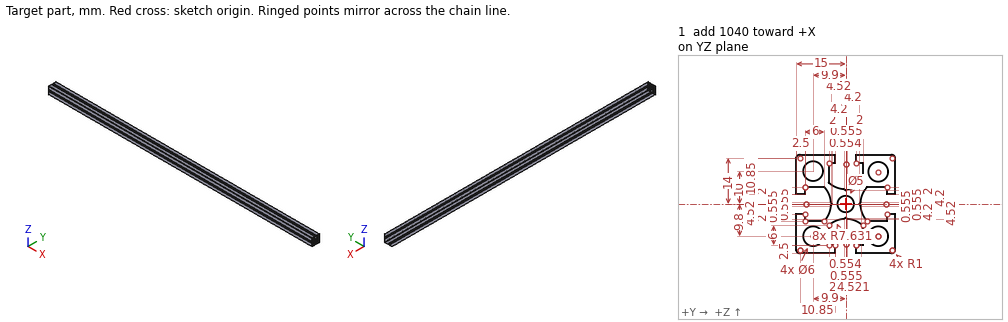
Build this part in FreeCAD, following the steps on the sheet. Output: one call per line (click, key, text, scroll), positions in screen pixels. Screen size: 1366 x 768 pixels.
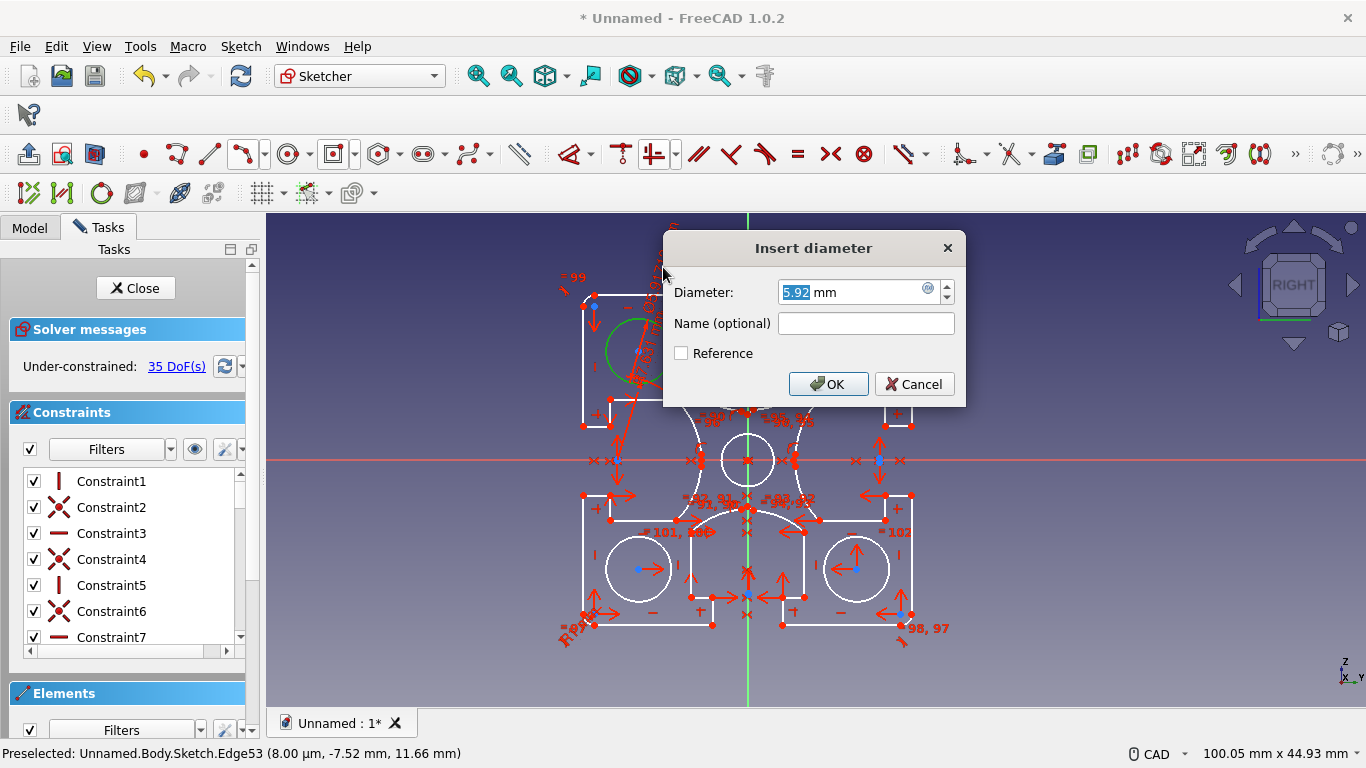
text(6)
key(Return)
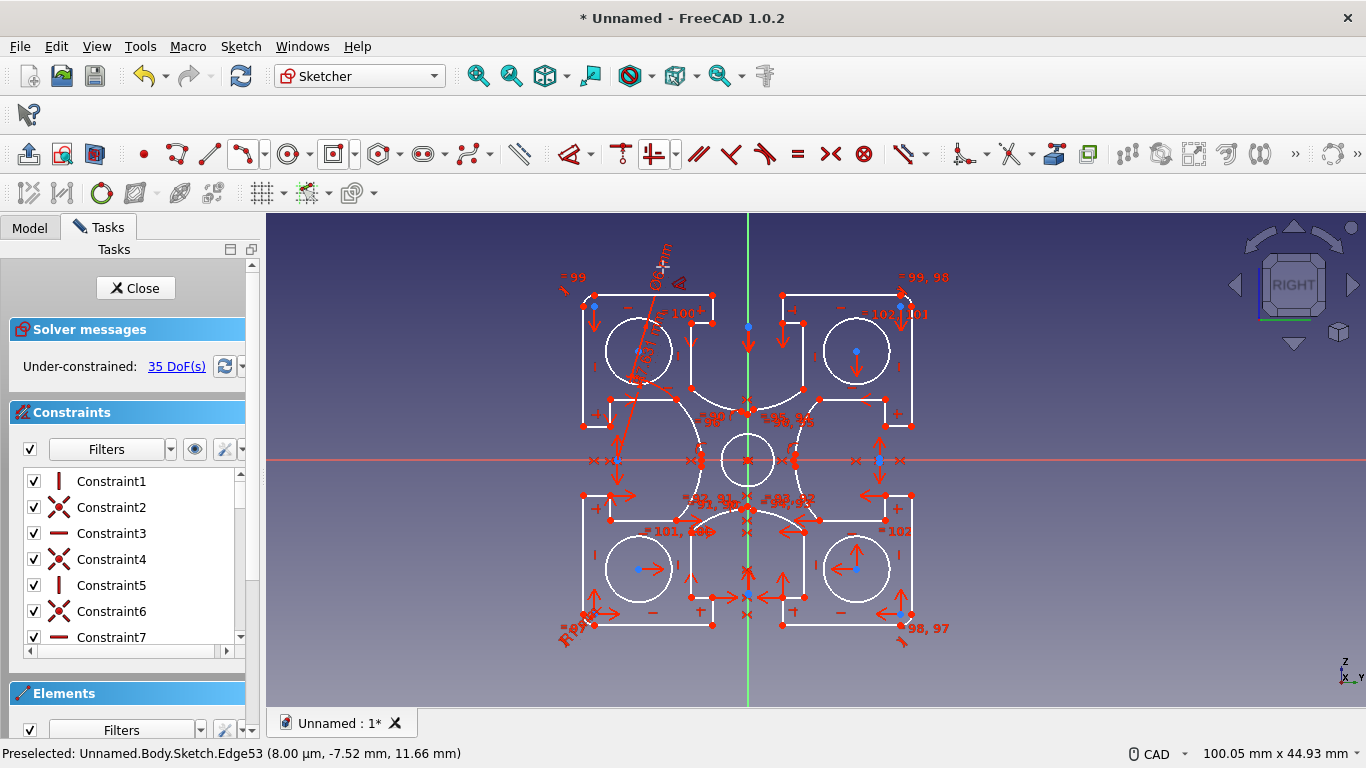
click(766, 442)
click(789, 419)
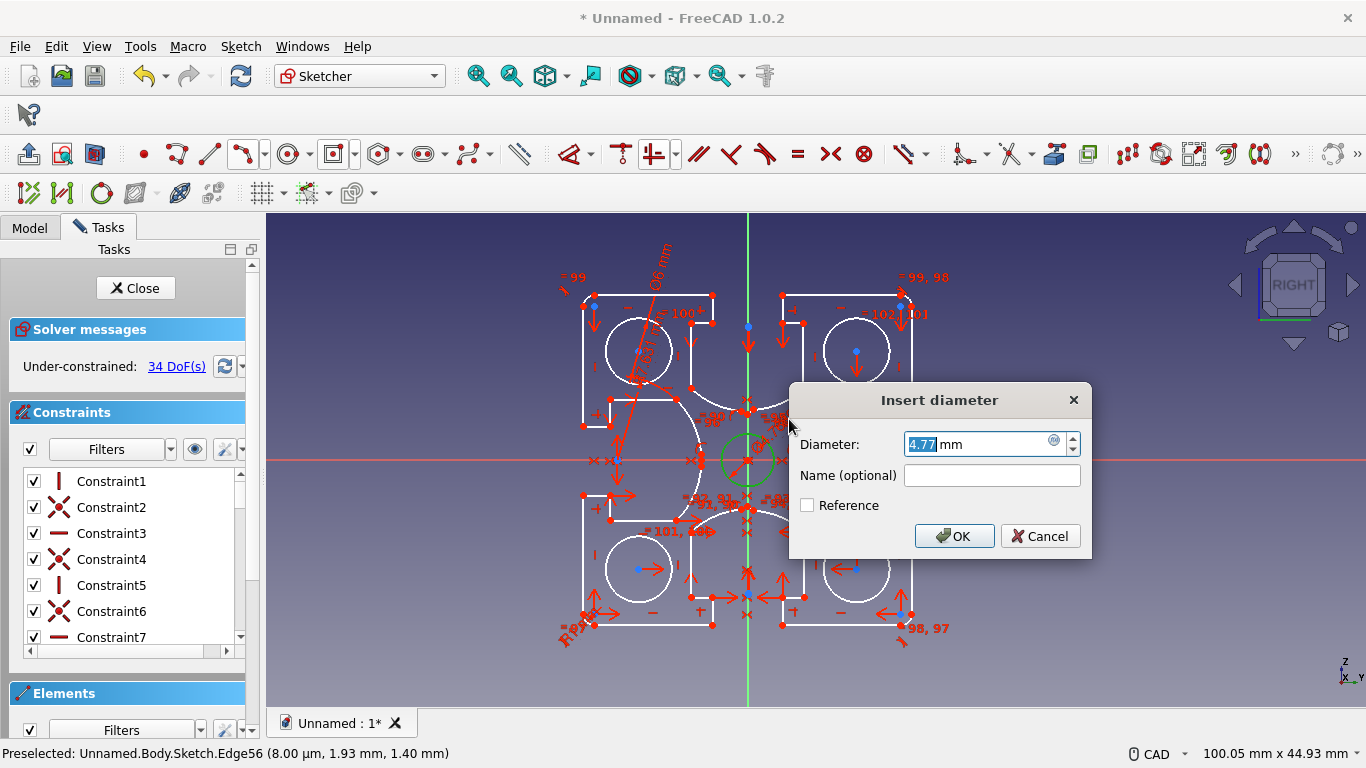
text(5)
key(Return)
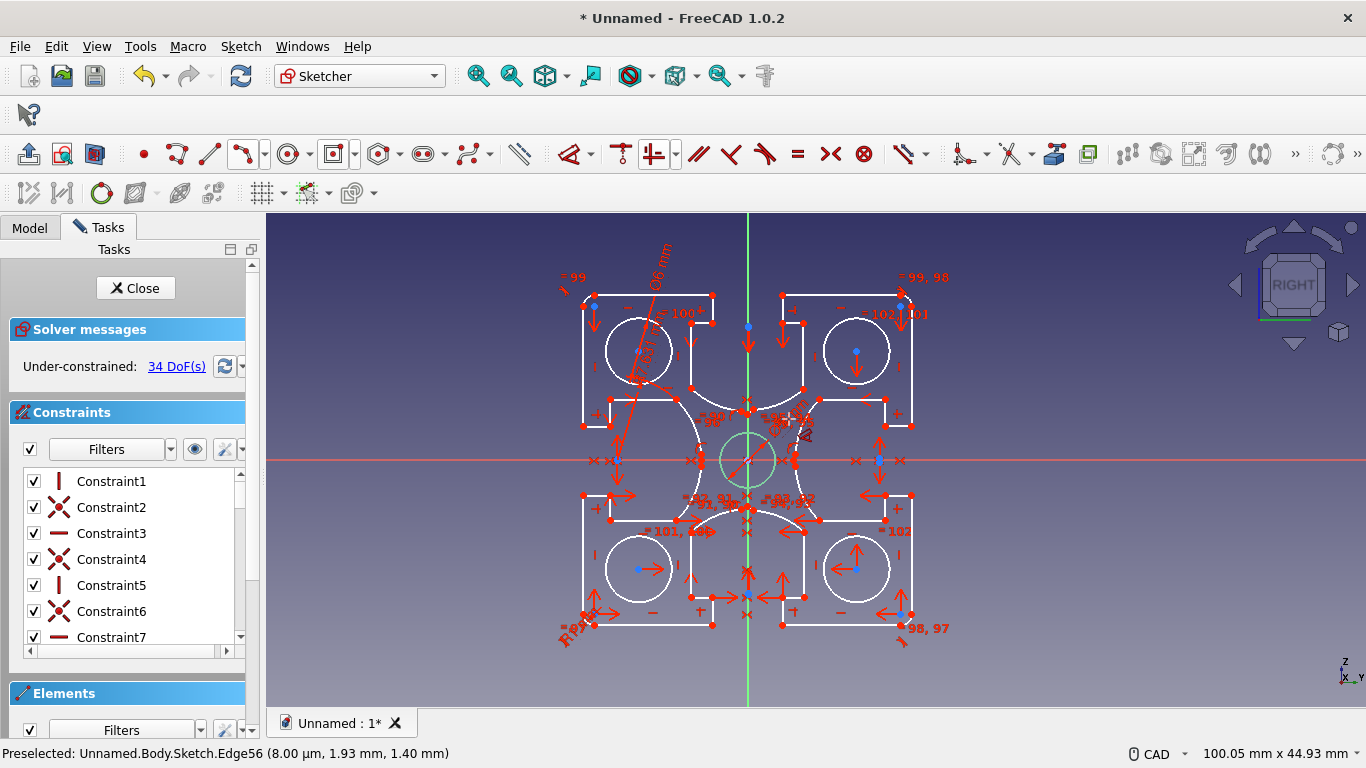
scroll(610, 416, up, 3)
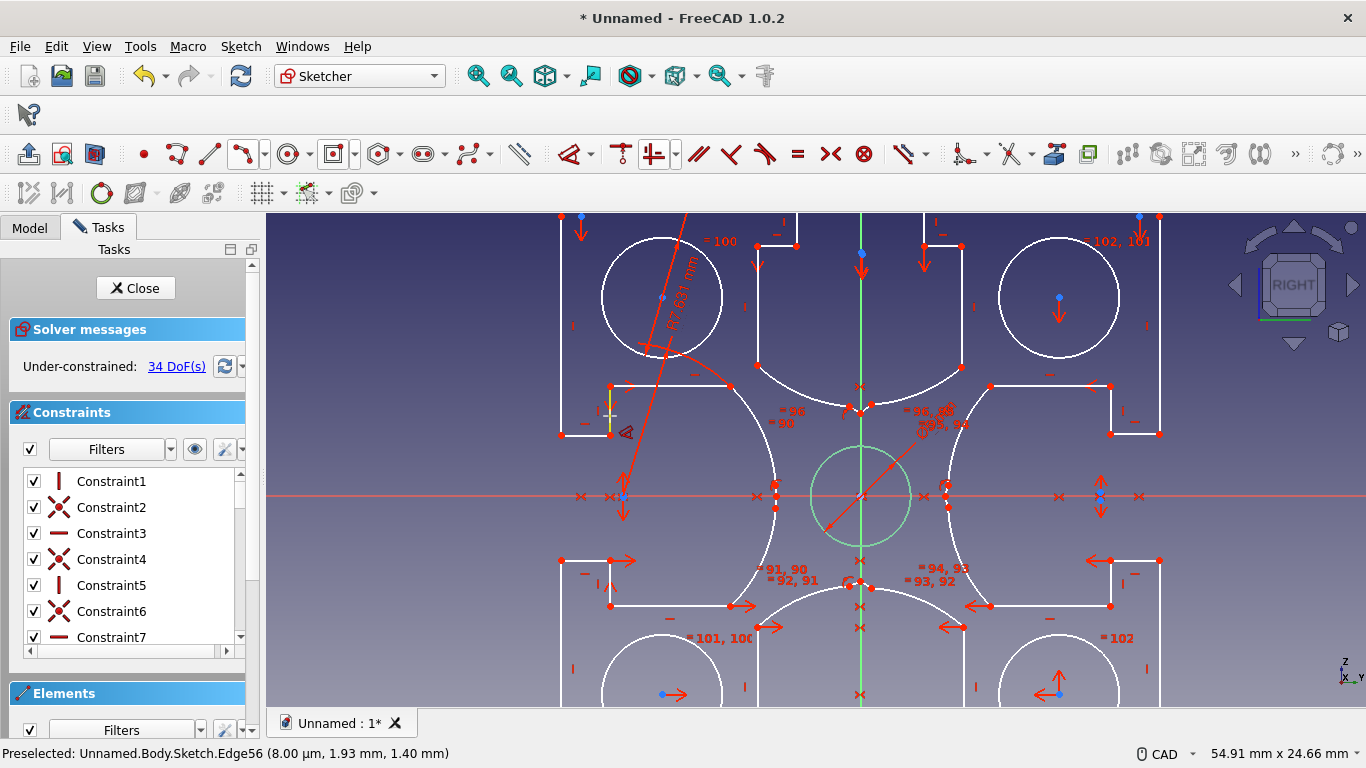
click(610, 416)
click(576, 411)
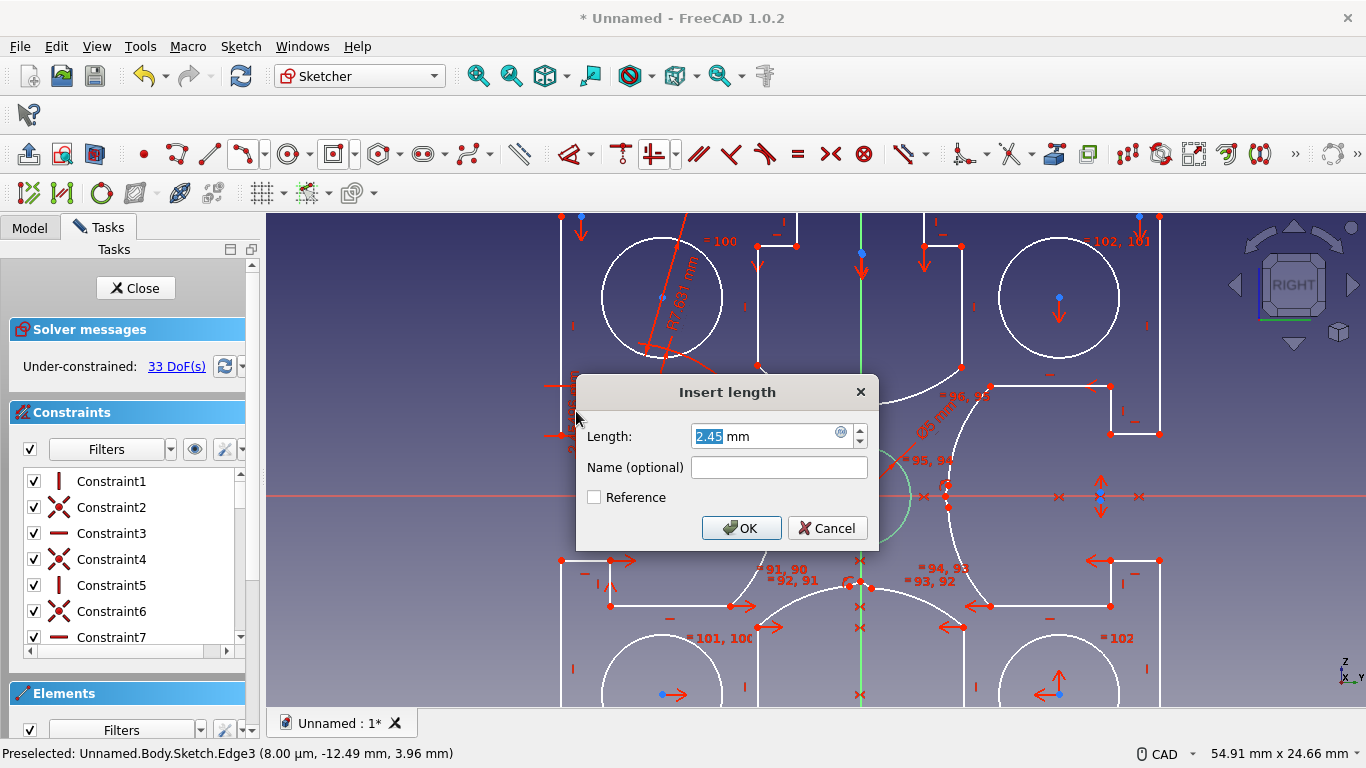
text(2)
key(Return)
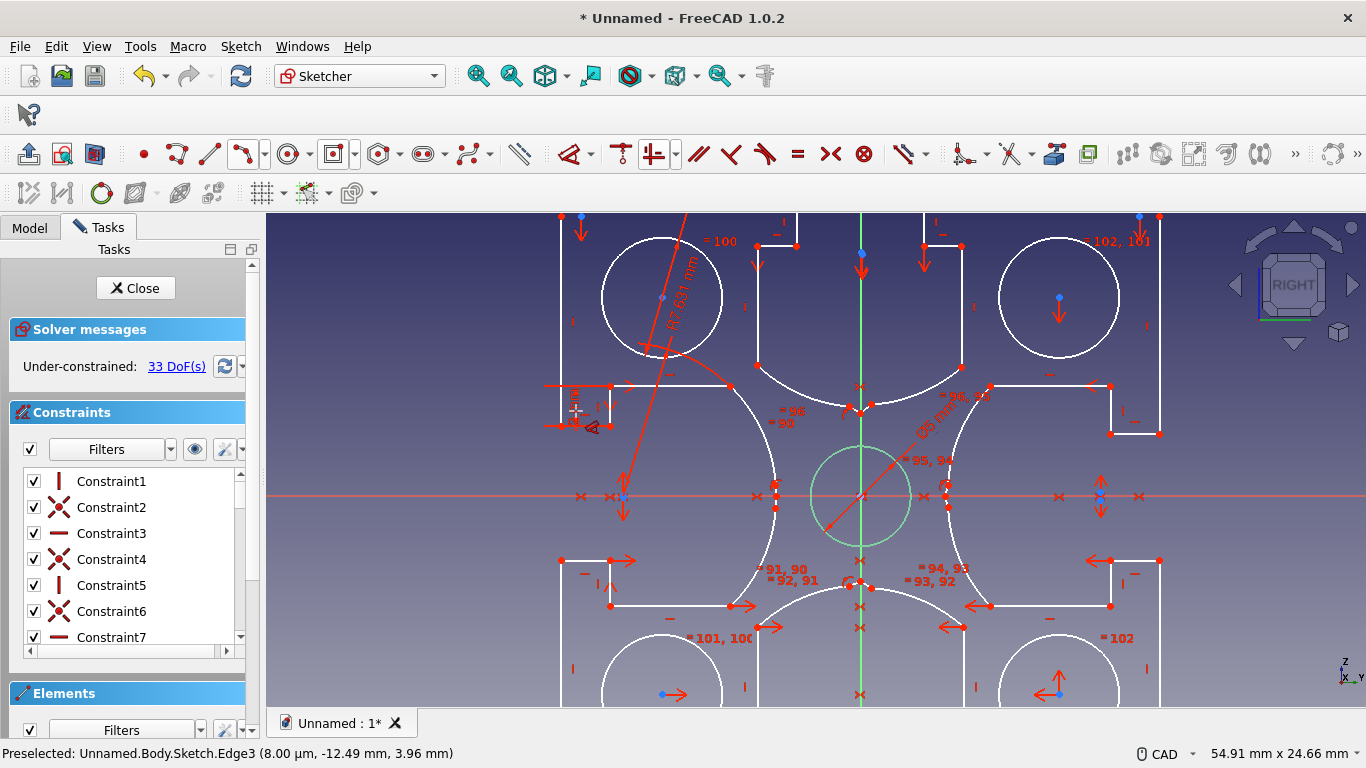
click(646, 386)
click(712, 352)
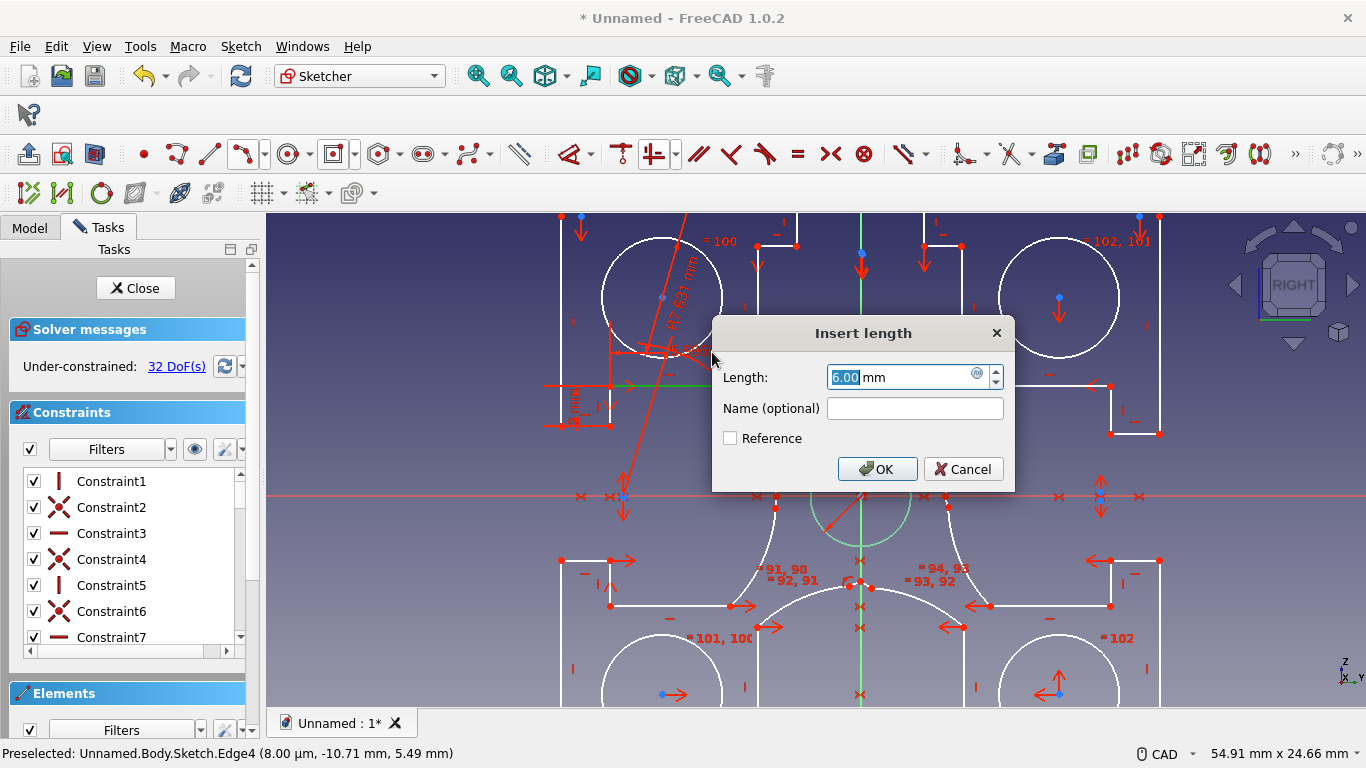
text(6)
key(Return)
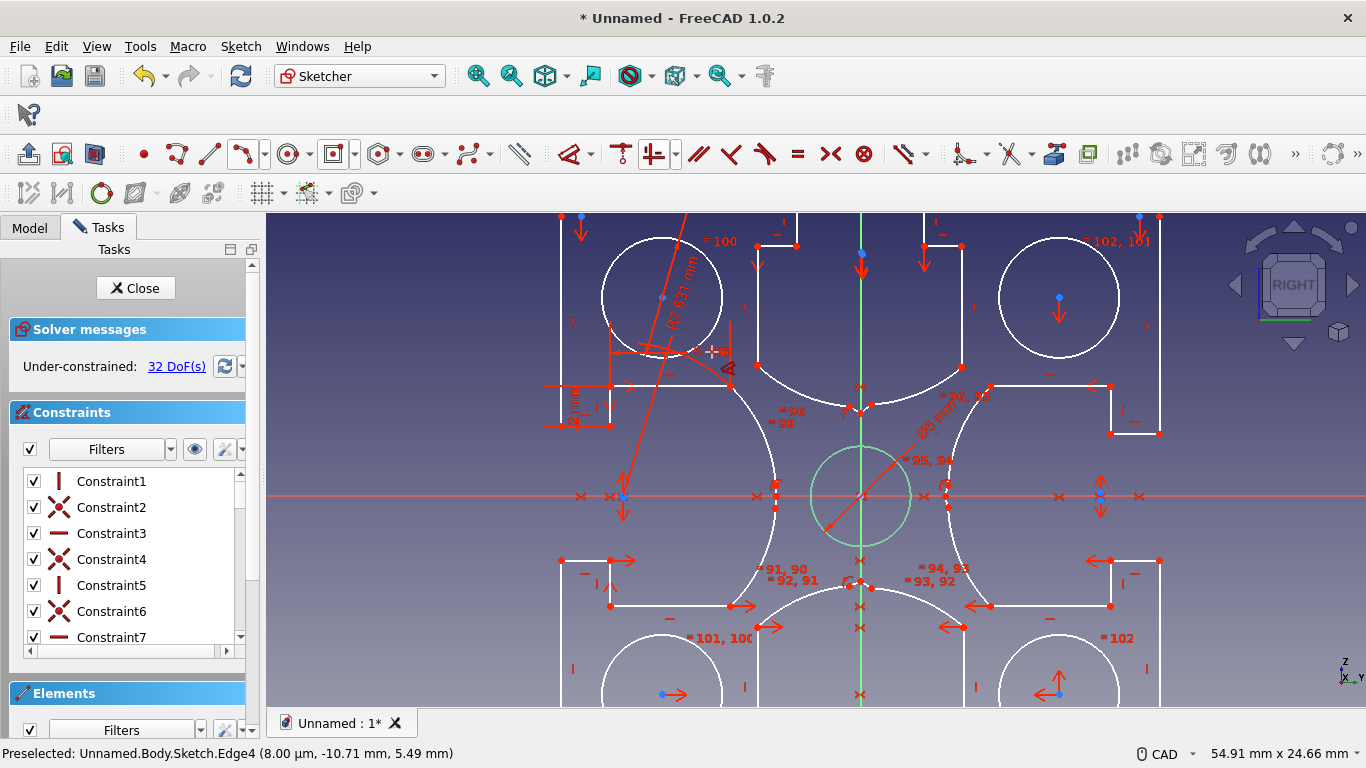
click(610, 593)
click(576, 584)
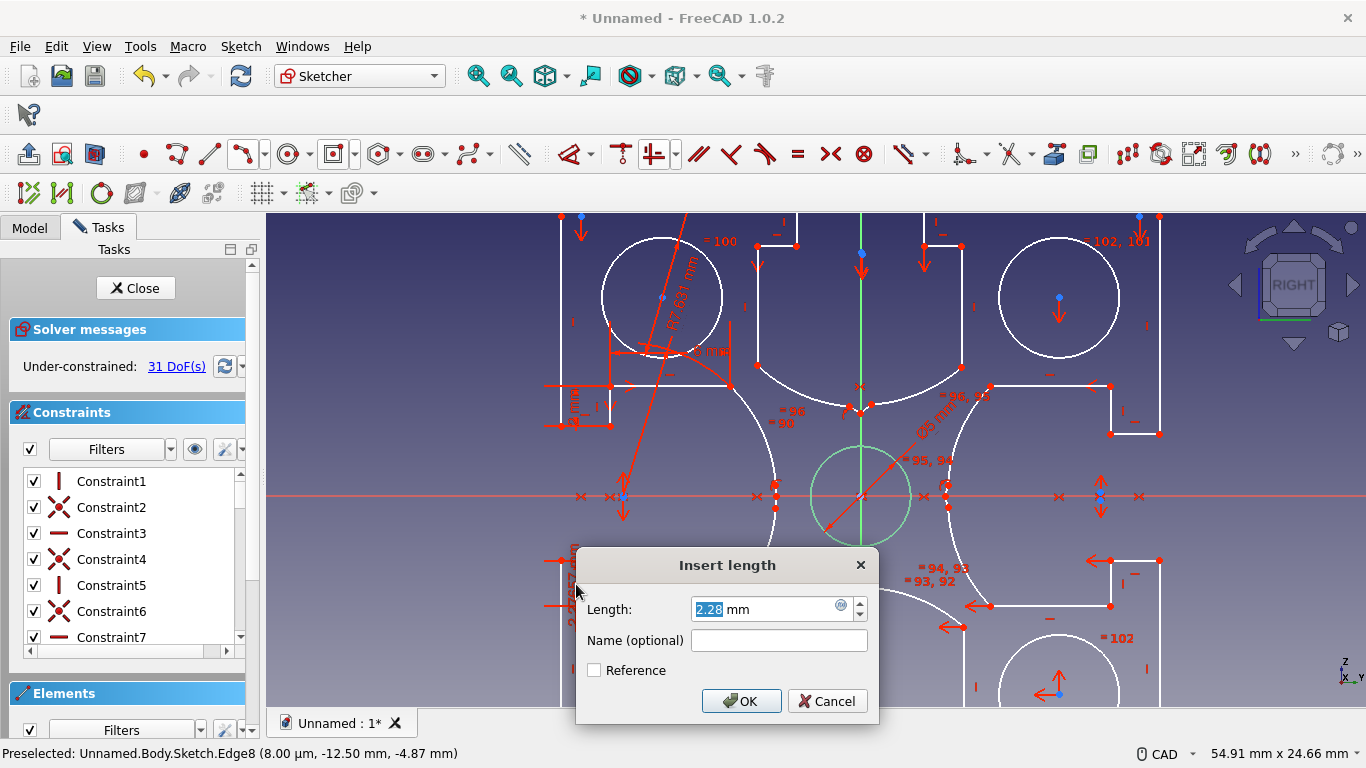
text(2)
key(Return)